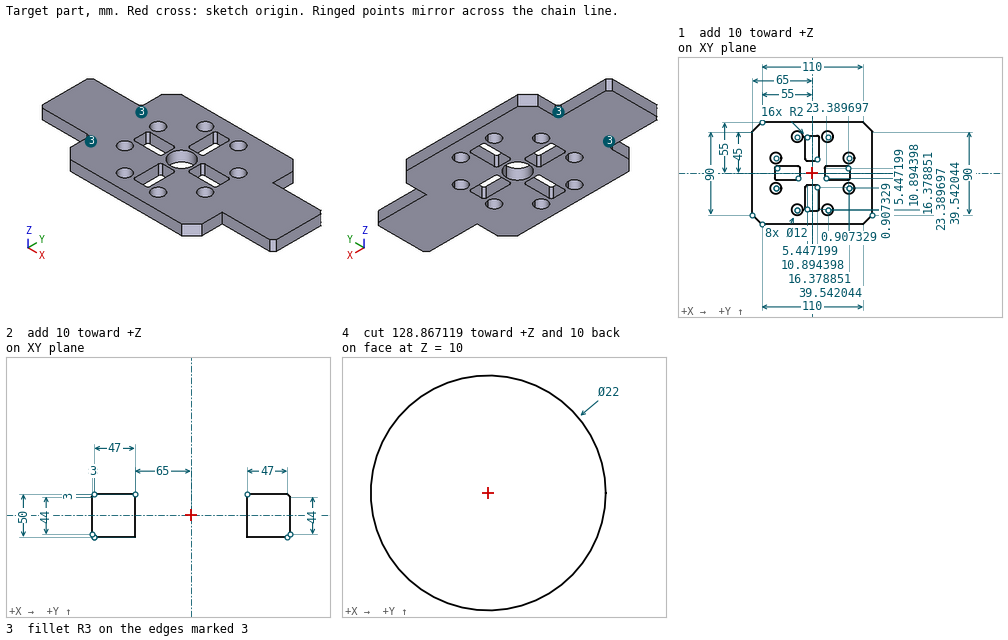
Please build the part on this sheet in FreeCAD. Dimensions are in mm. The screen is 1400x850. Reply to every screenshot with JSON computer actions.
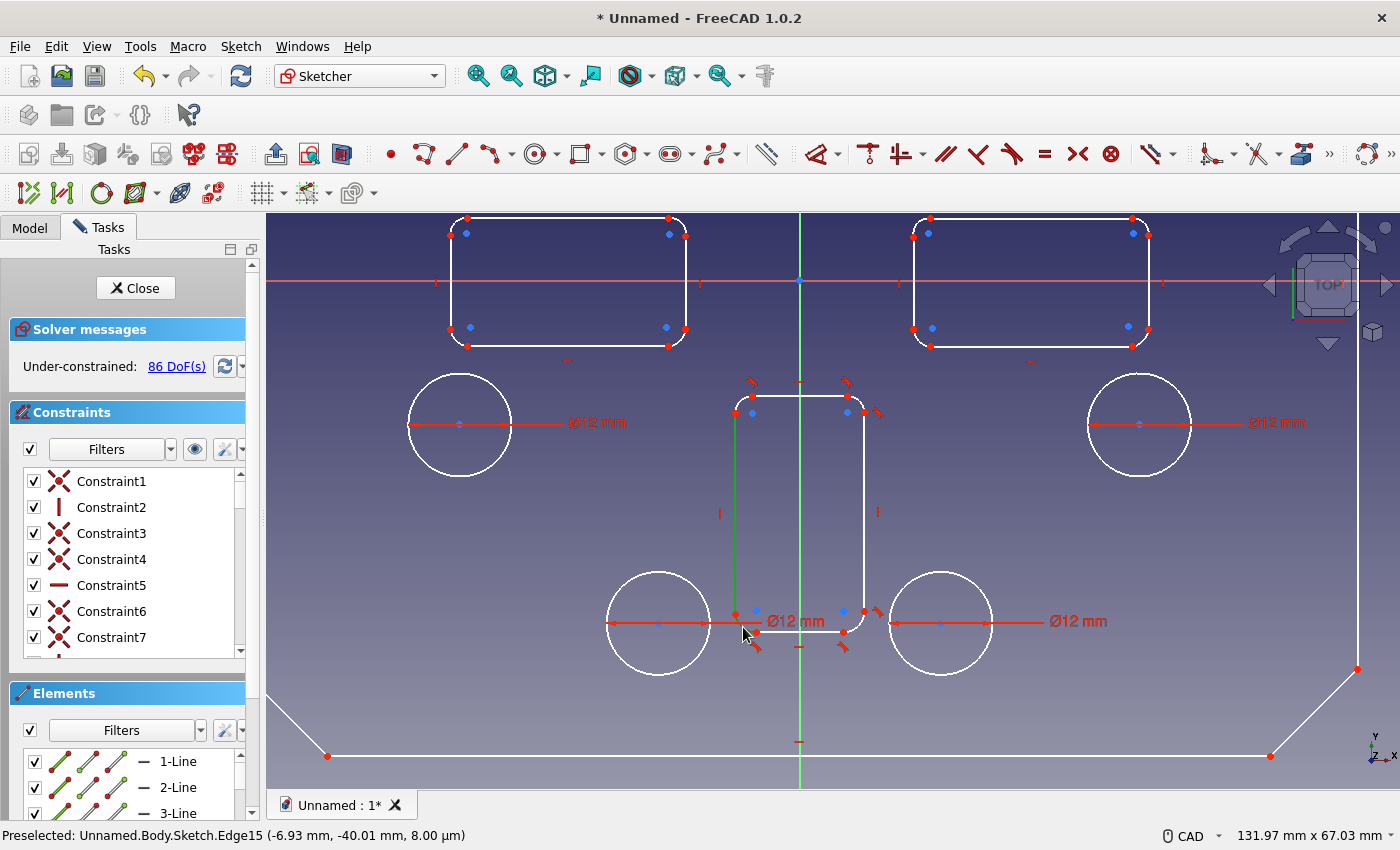
{"action": "left_click", "coordinate": [1012, 154]}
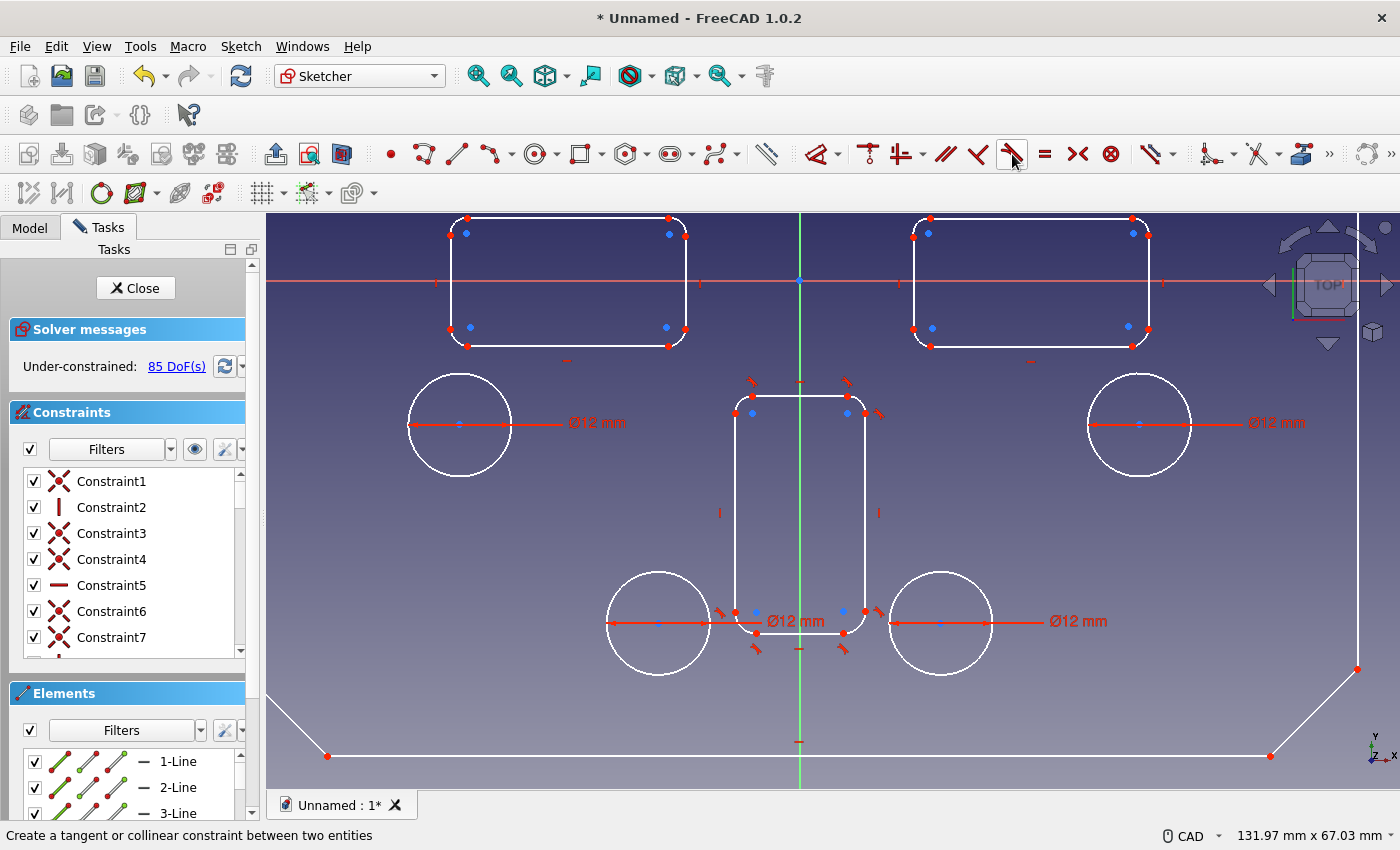
{"action": "left_click", "coordinate": [735, 552]}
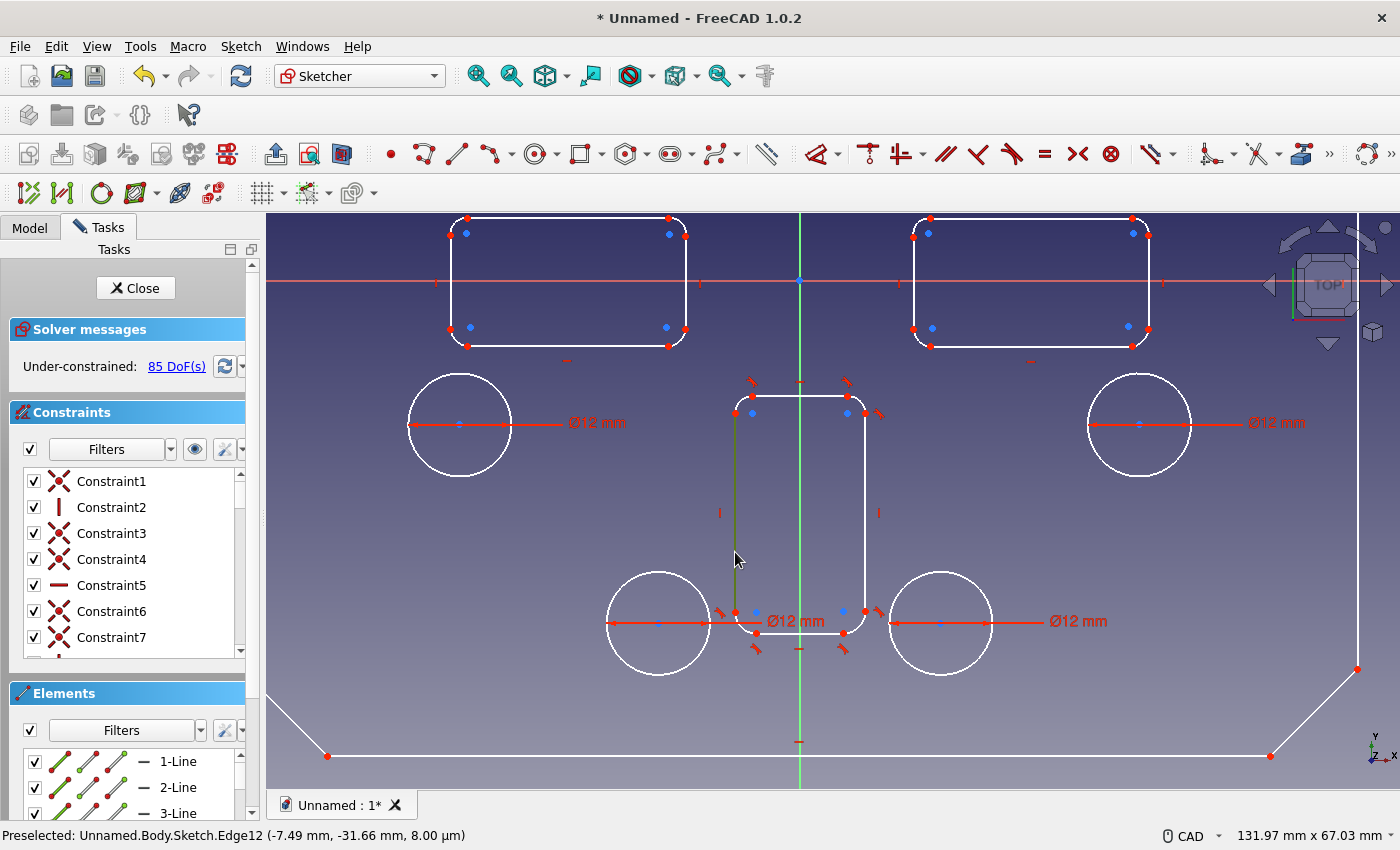
{"action": "left_click", "coordinate": [740, 401]}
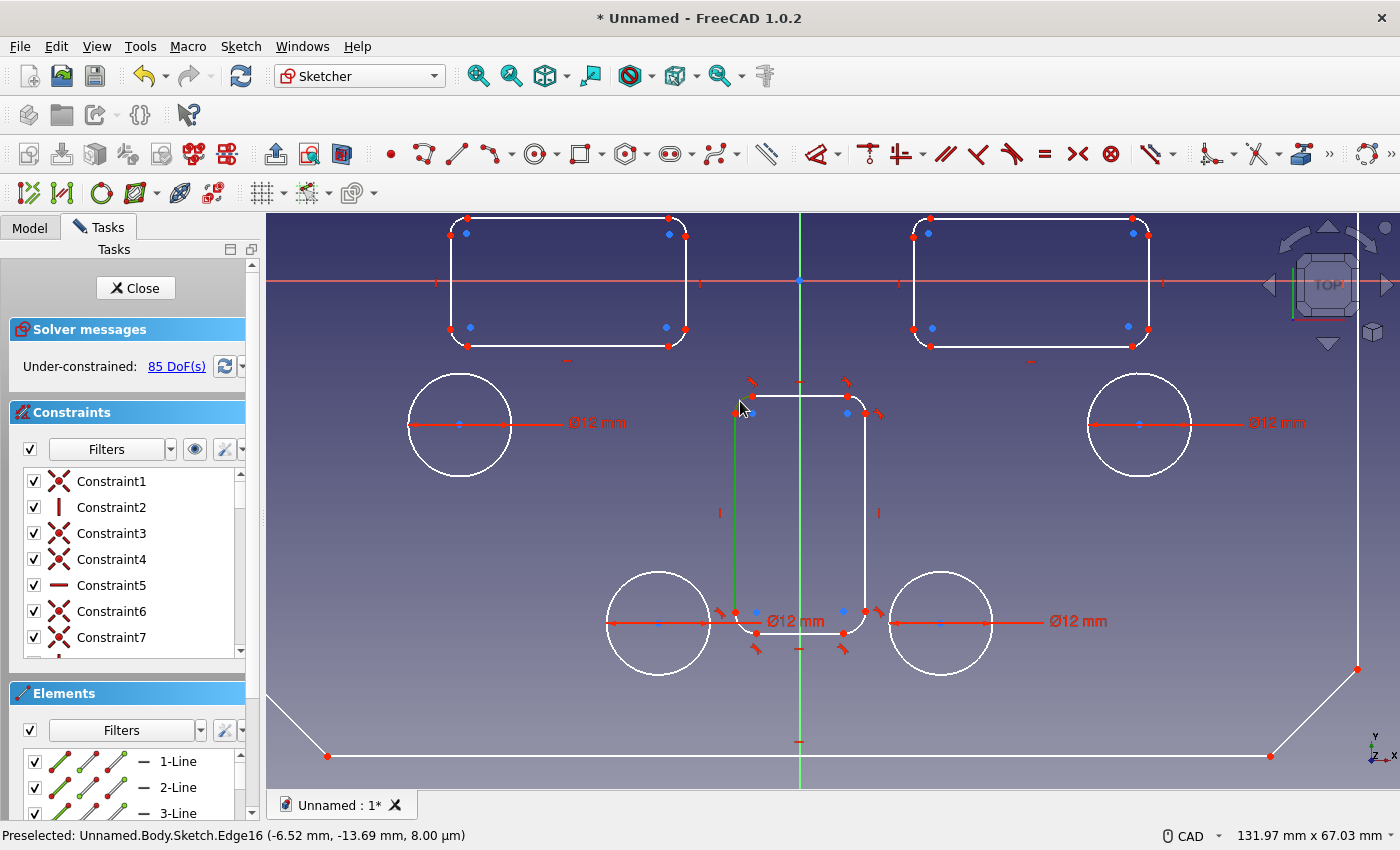
{"action": "left_click", "coordinate": [1012, 154]}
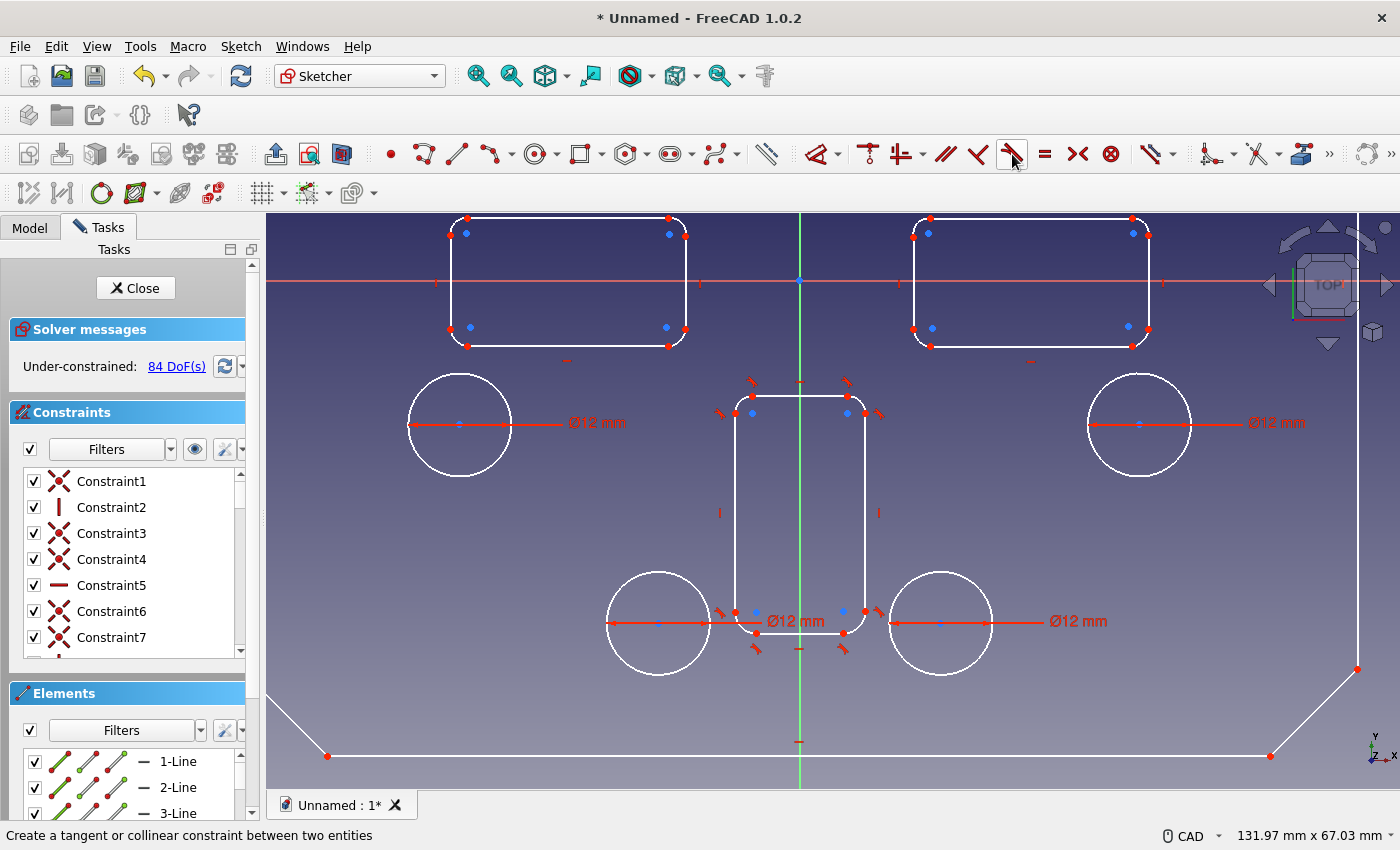
{"action": "left_click", "coordinate": [914, 302]}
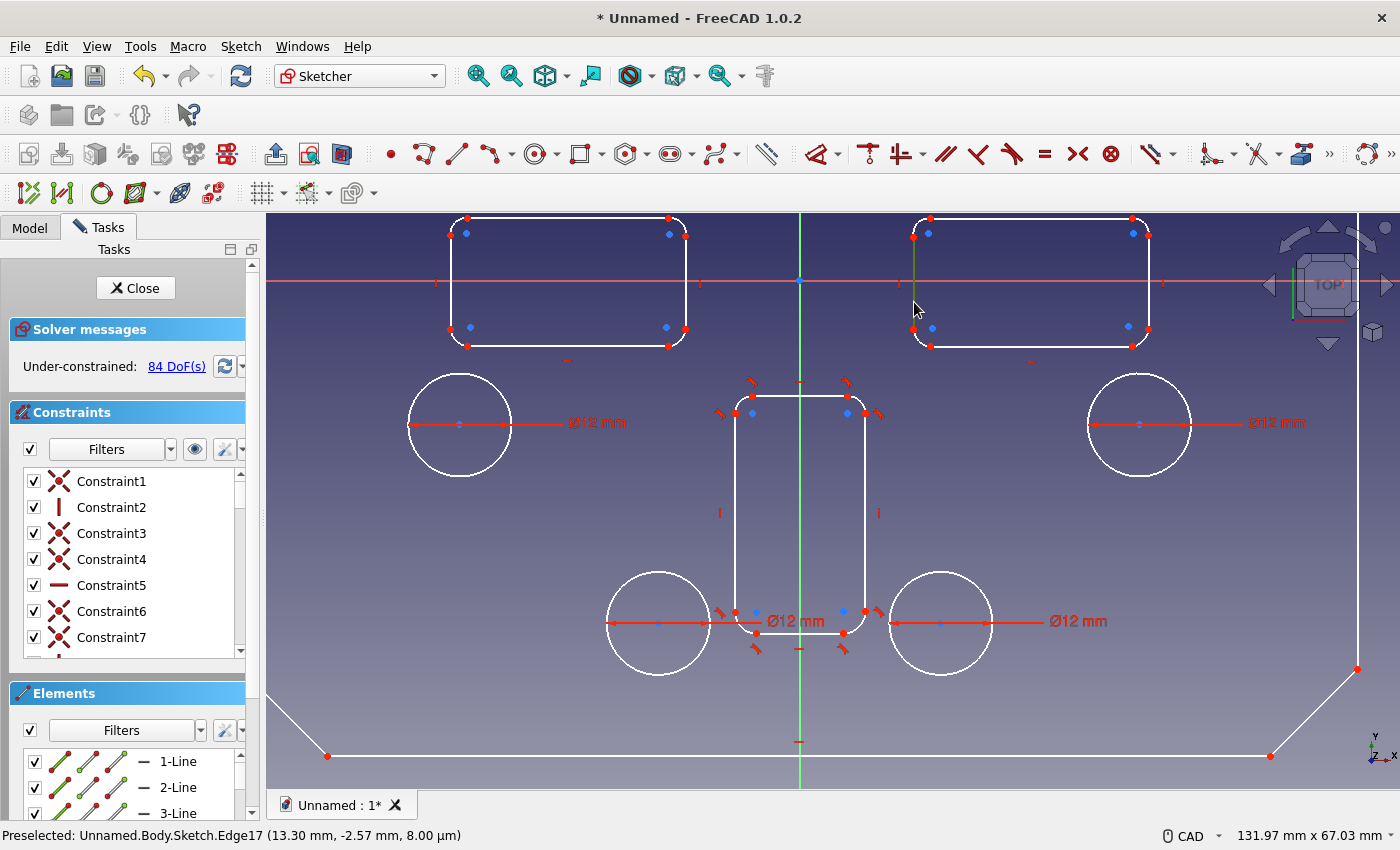
{"action": "scroll", "coordinate": [744, 629], "scroll_direction": "down", "scroll_amount": 5}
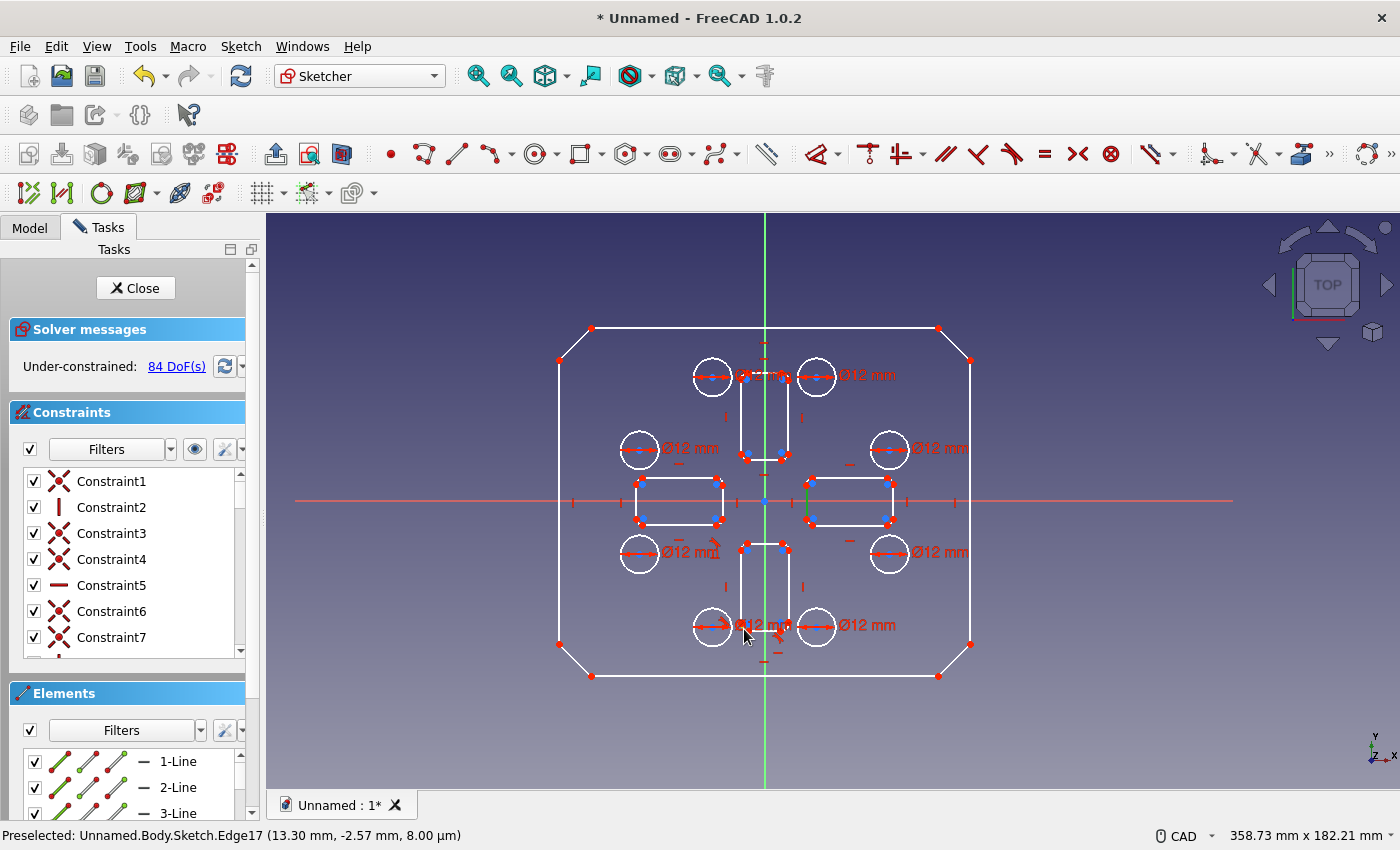
{"action": "scroll", "coordinate": [808, 480], "scroll_direction": "up", "scroll_amount": 5}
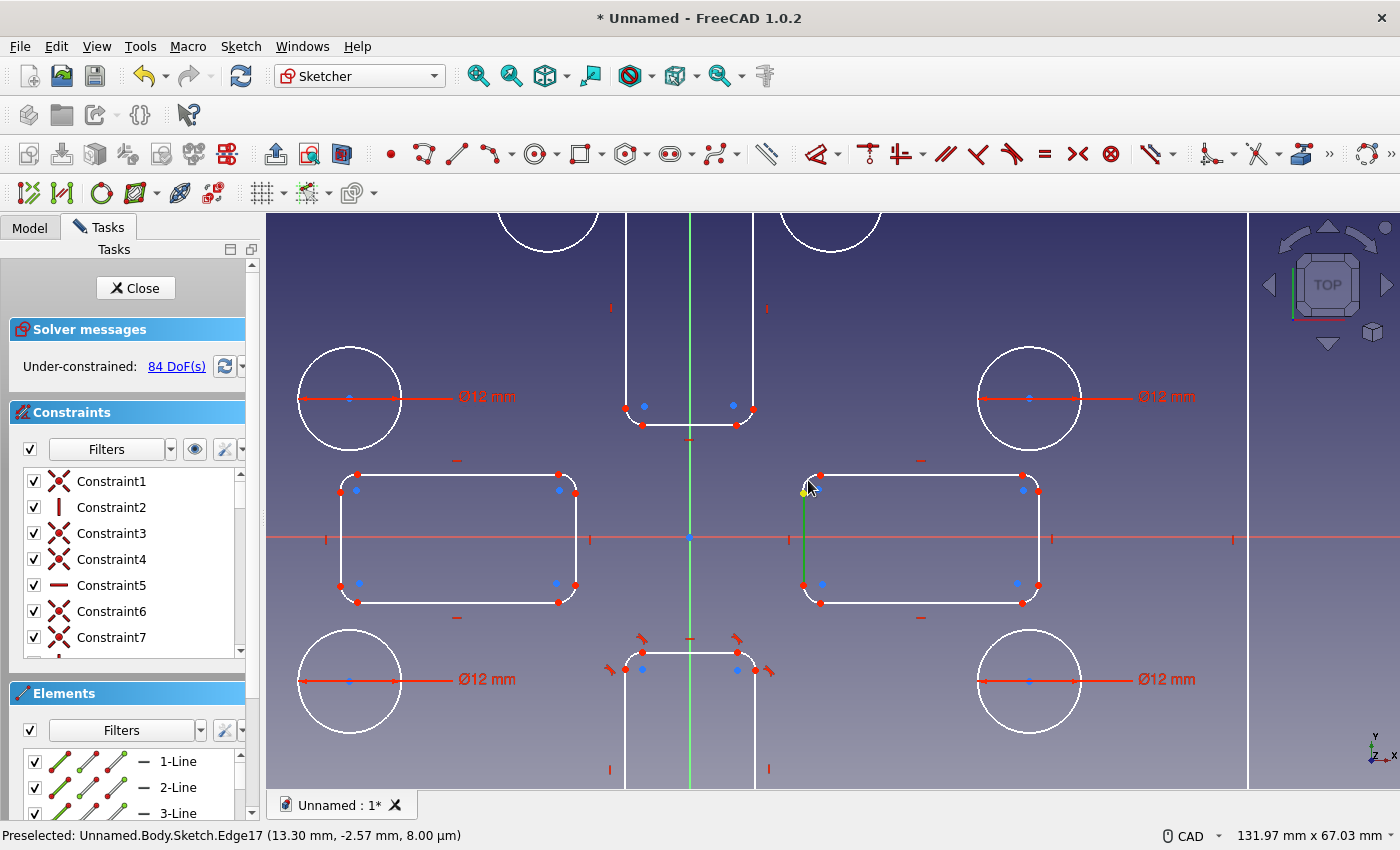
{"action": "left_click", "coordinate": [807, 480]}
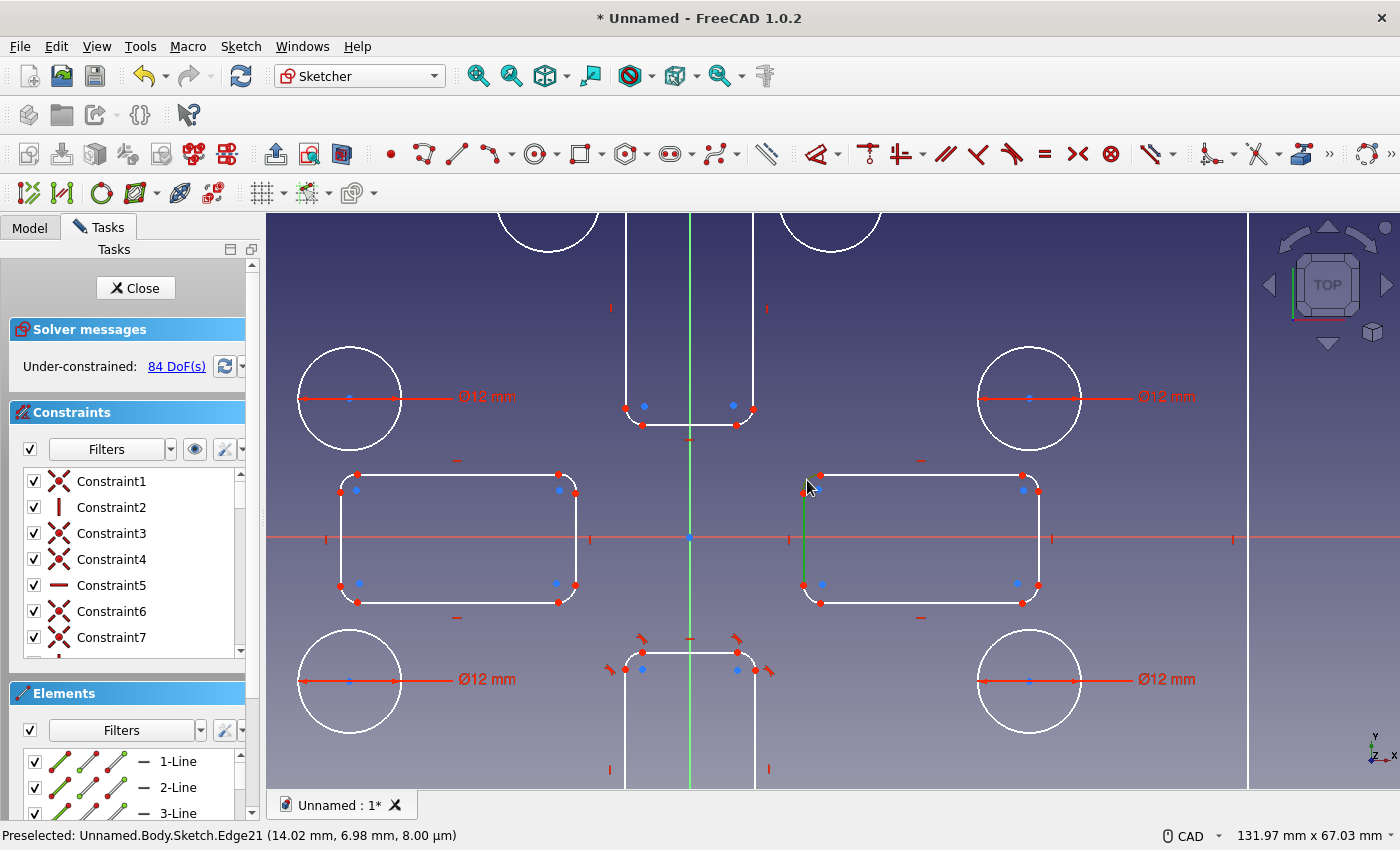
{"action": "left_click", "coordinate": [1012, 154]}